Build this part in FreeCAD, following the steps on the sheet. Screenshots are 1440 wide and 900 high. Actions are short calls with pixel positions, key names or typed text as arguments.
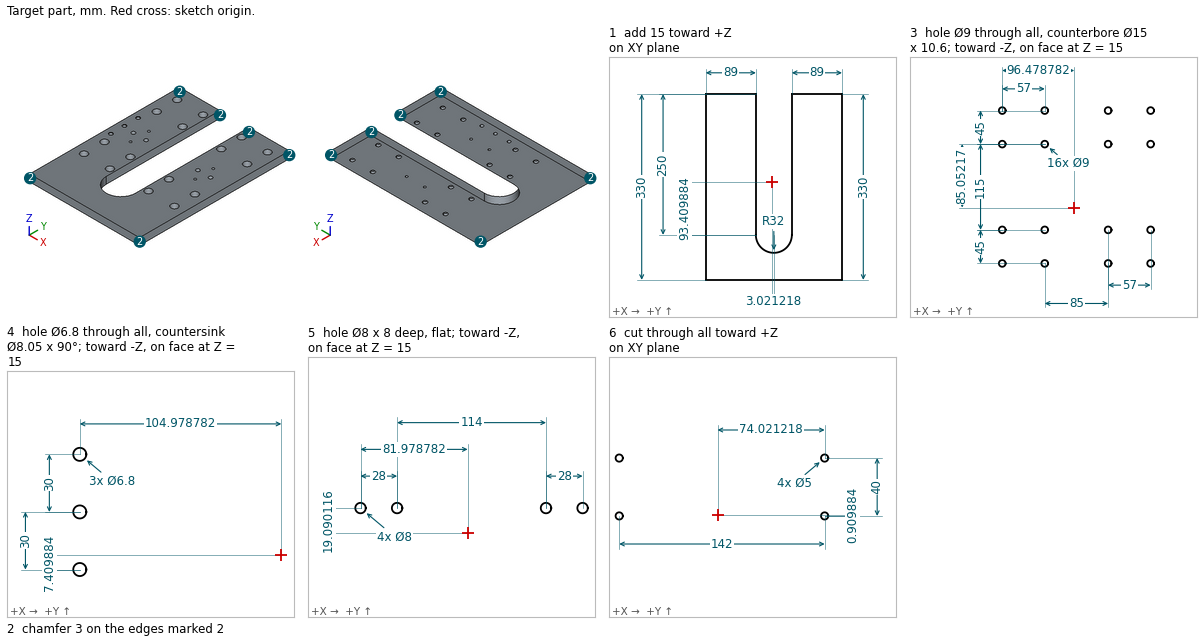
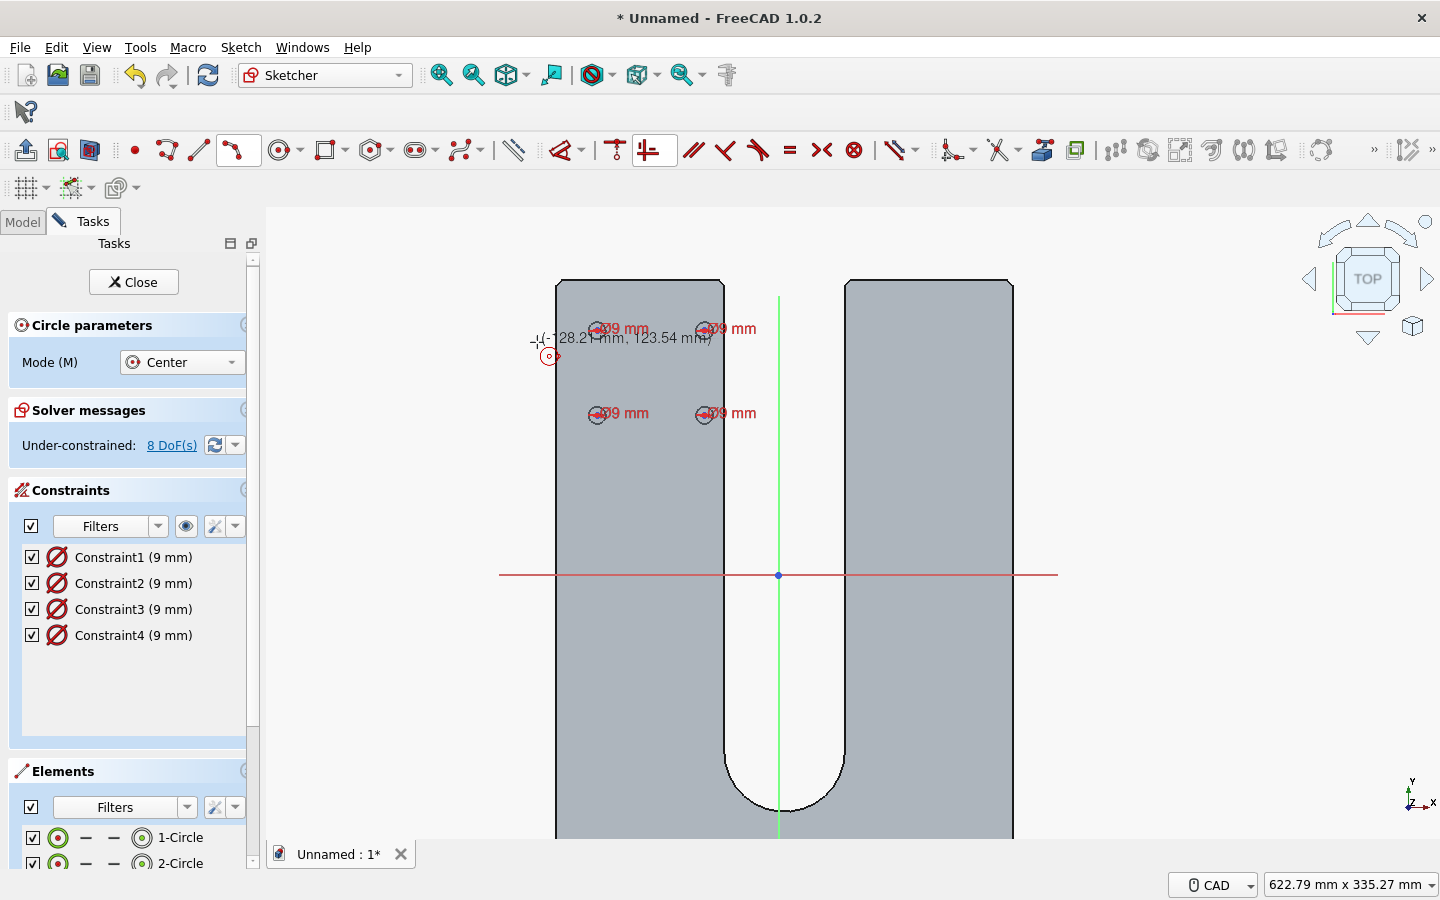
scroll(597, 632, up, 5)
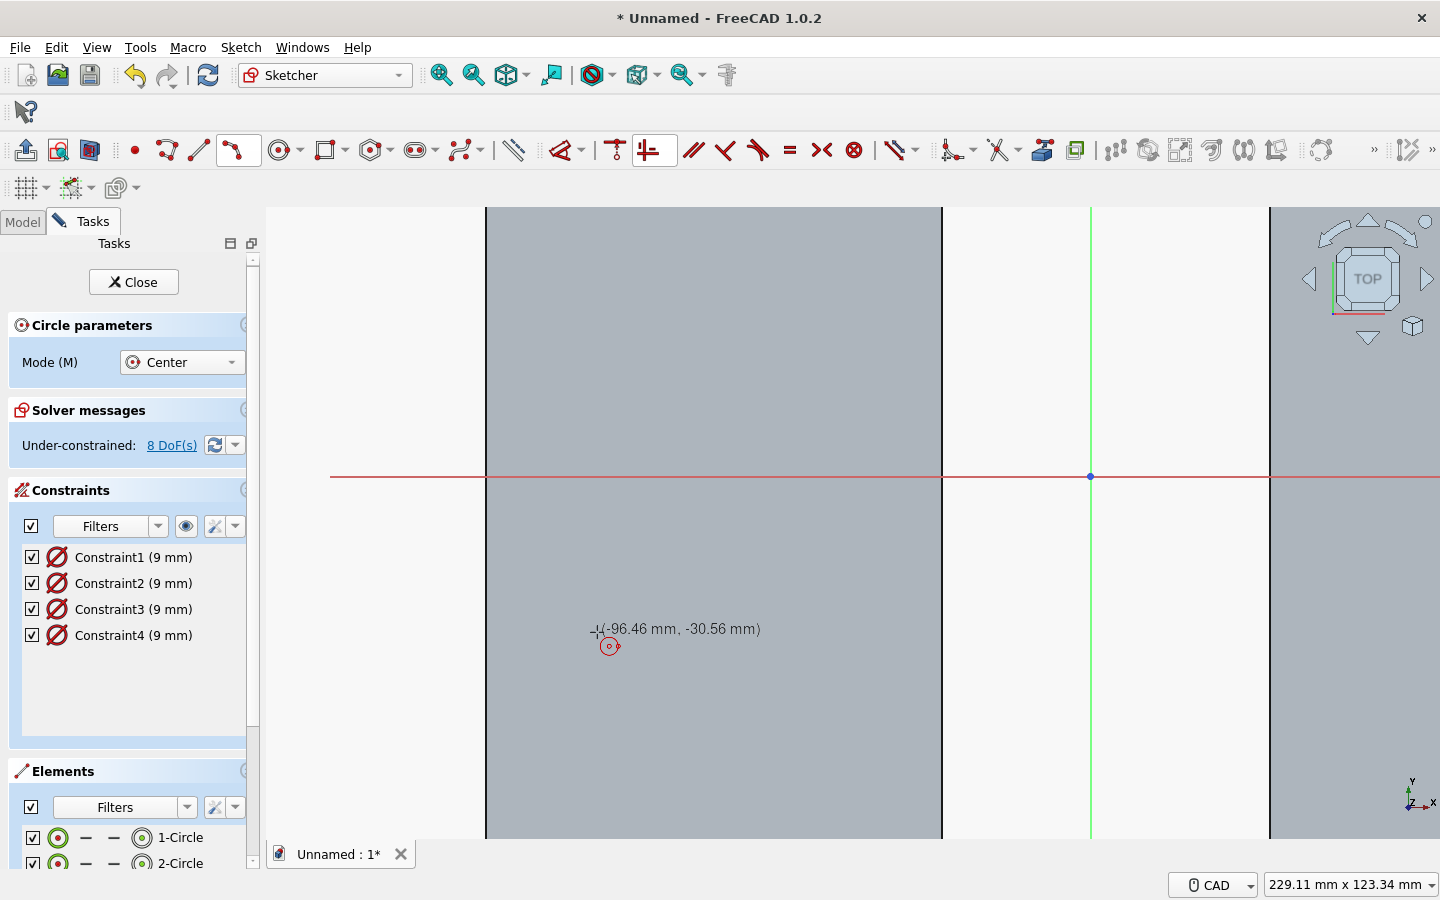
click(596, 630)
move(613, 614)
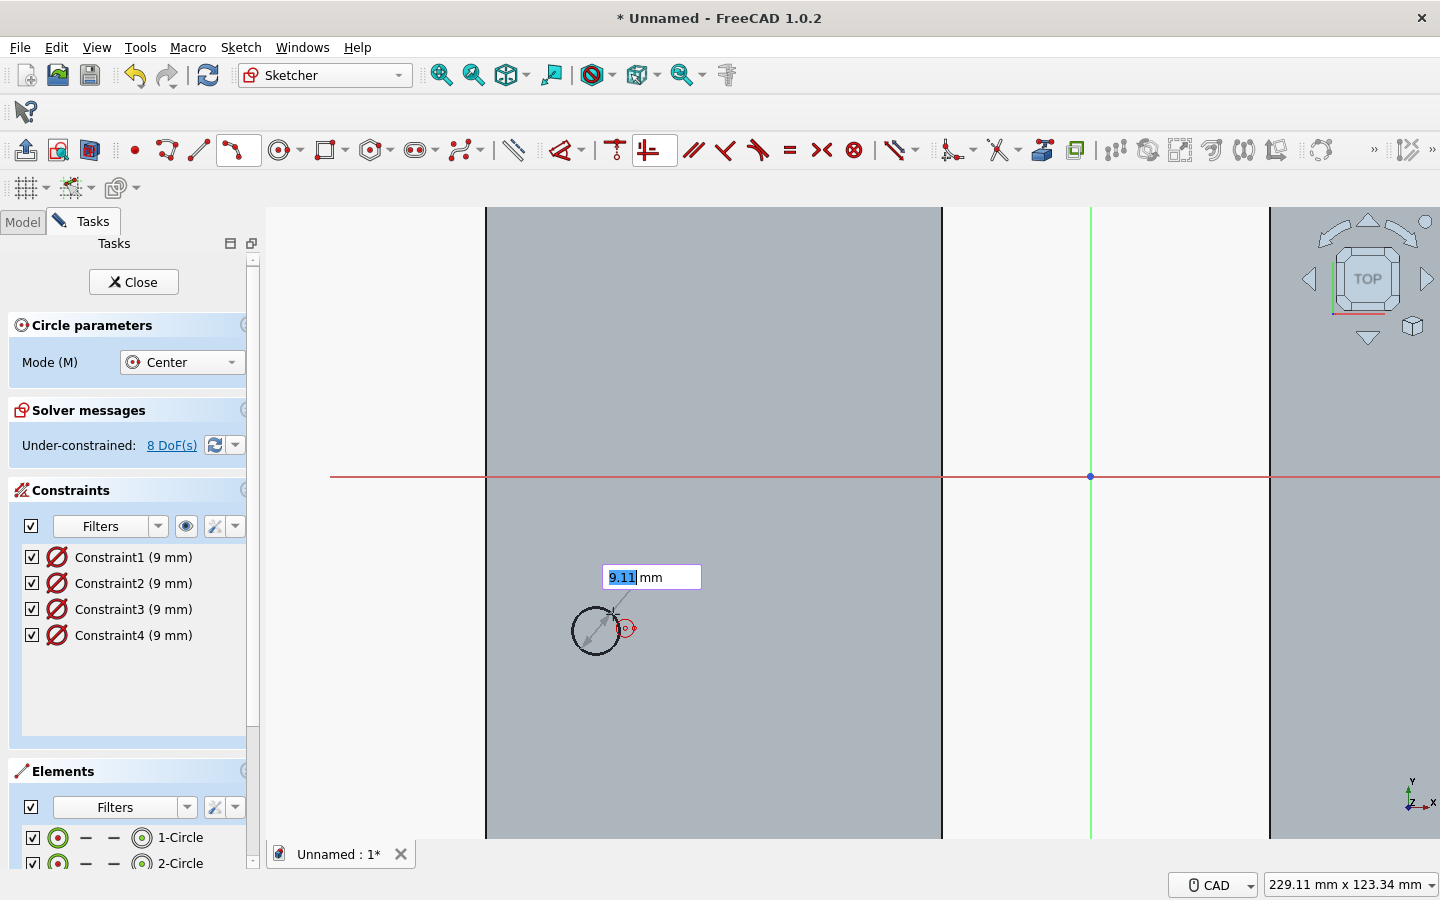
text(9)
key(Return)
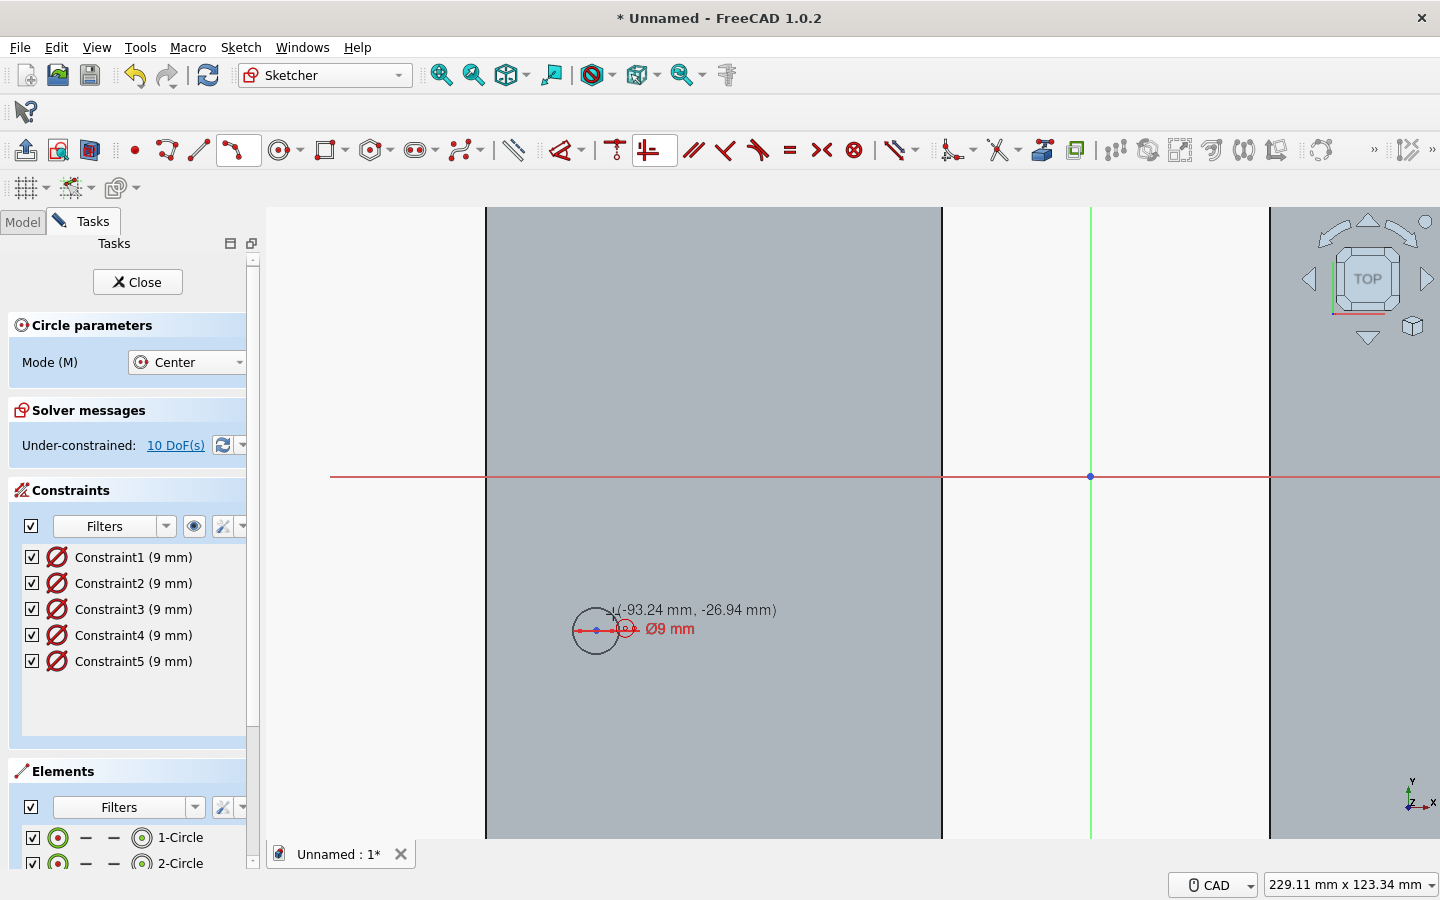
click(888, 630)
move(905, 614)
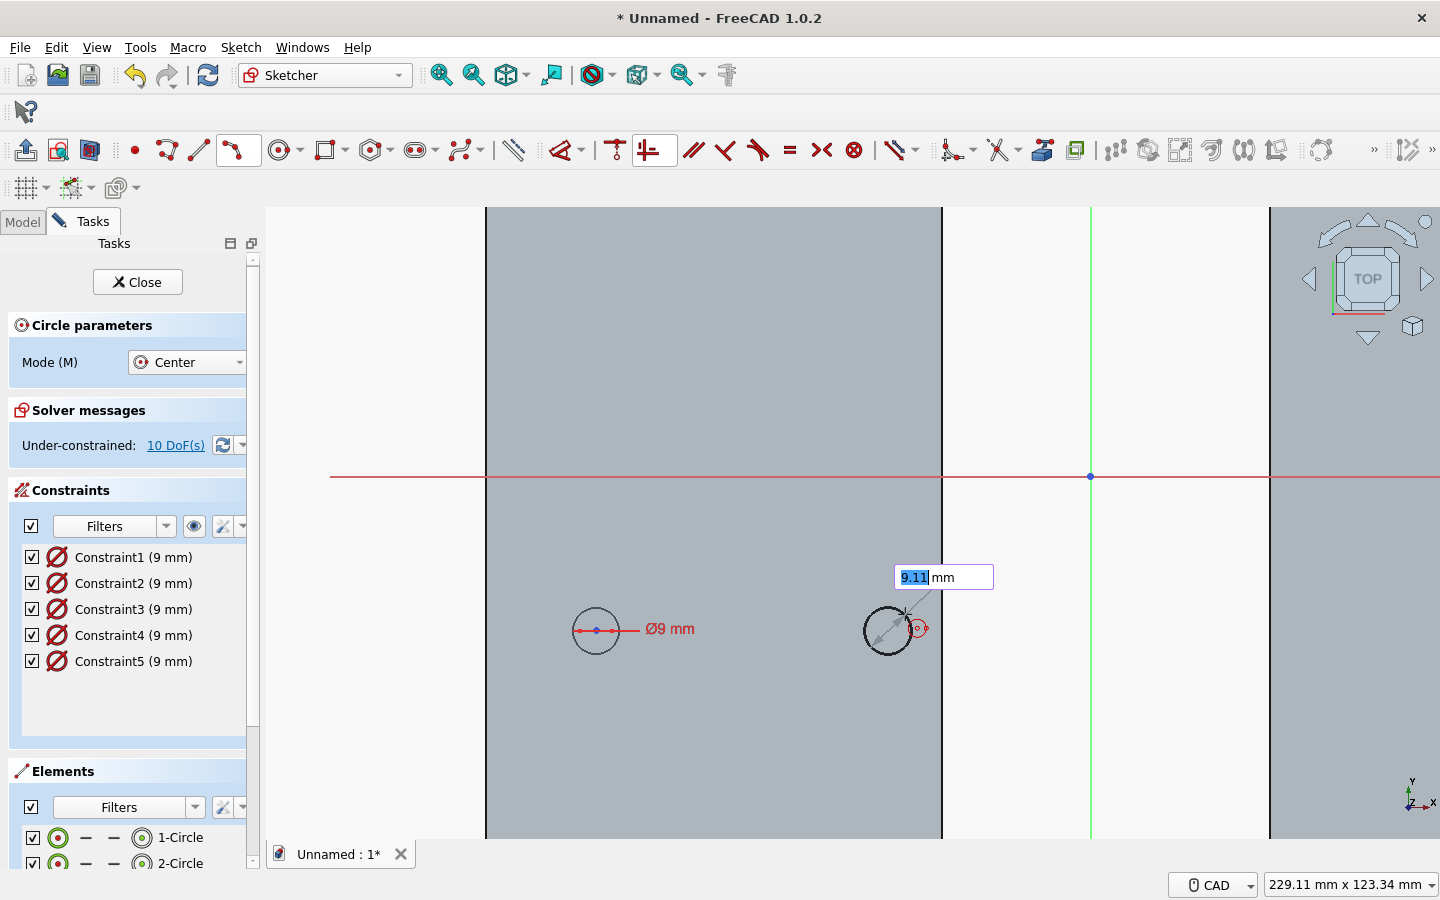
text(9)
key(Return)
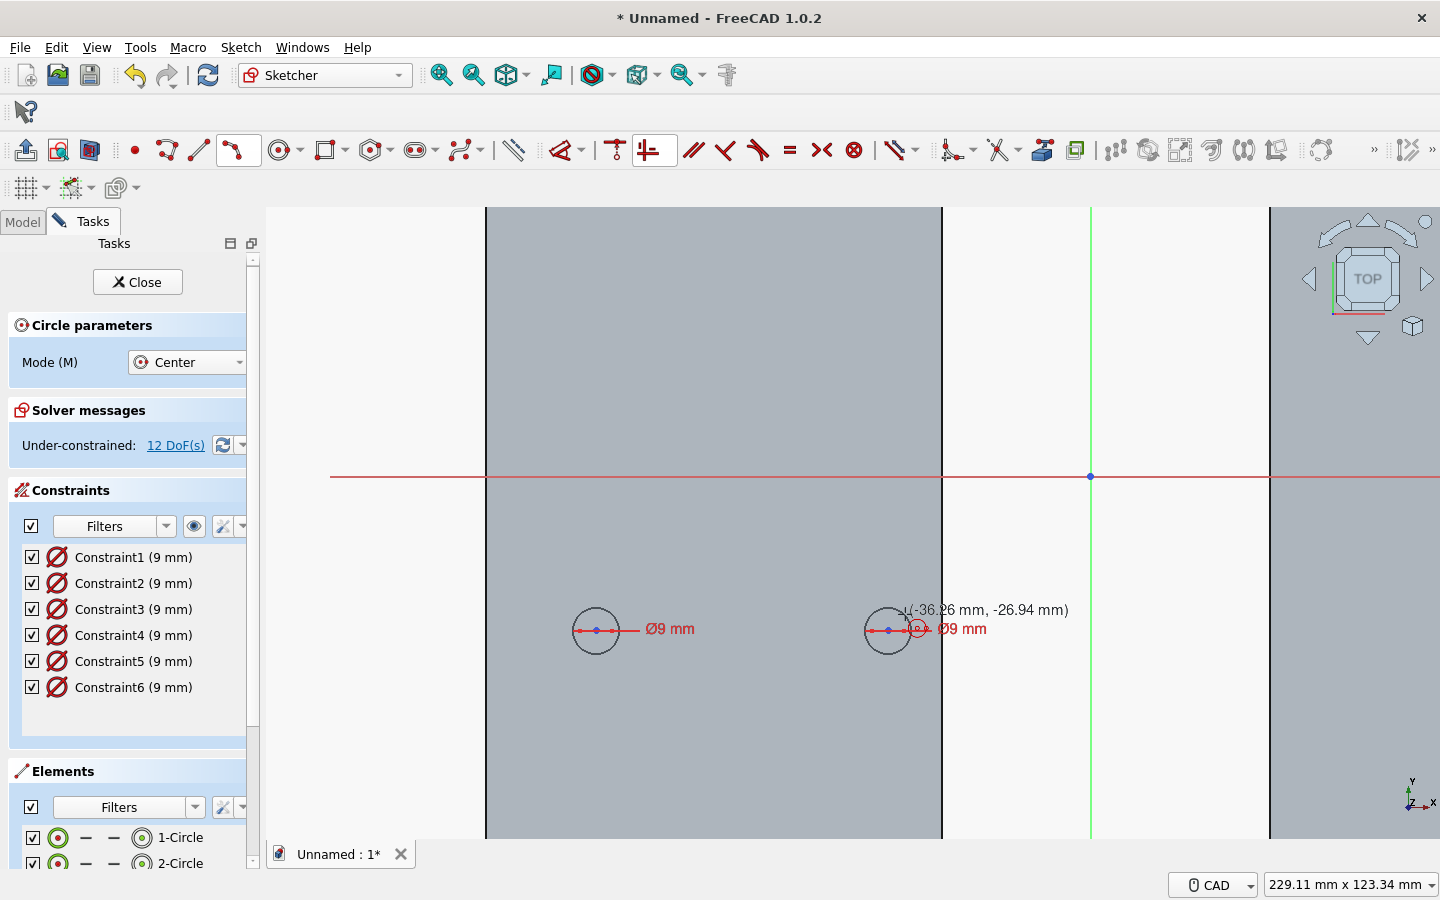
scroll(597, 632, down, 5)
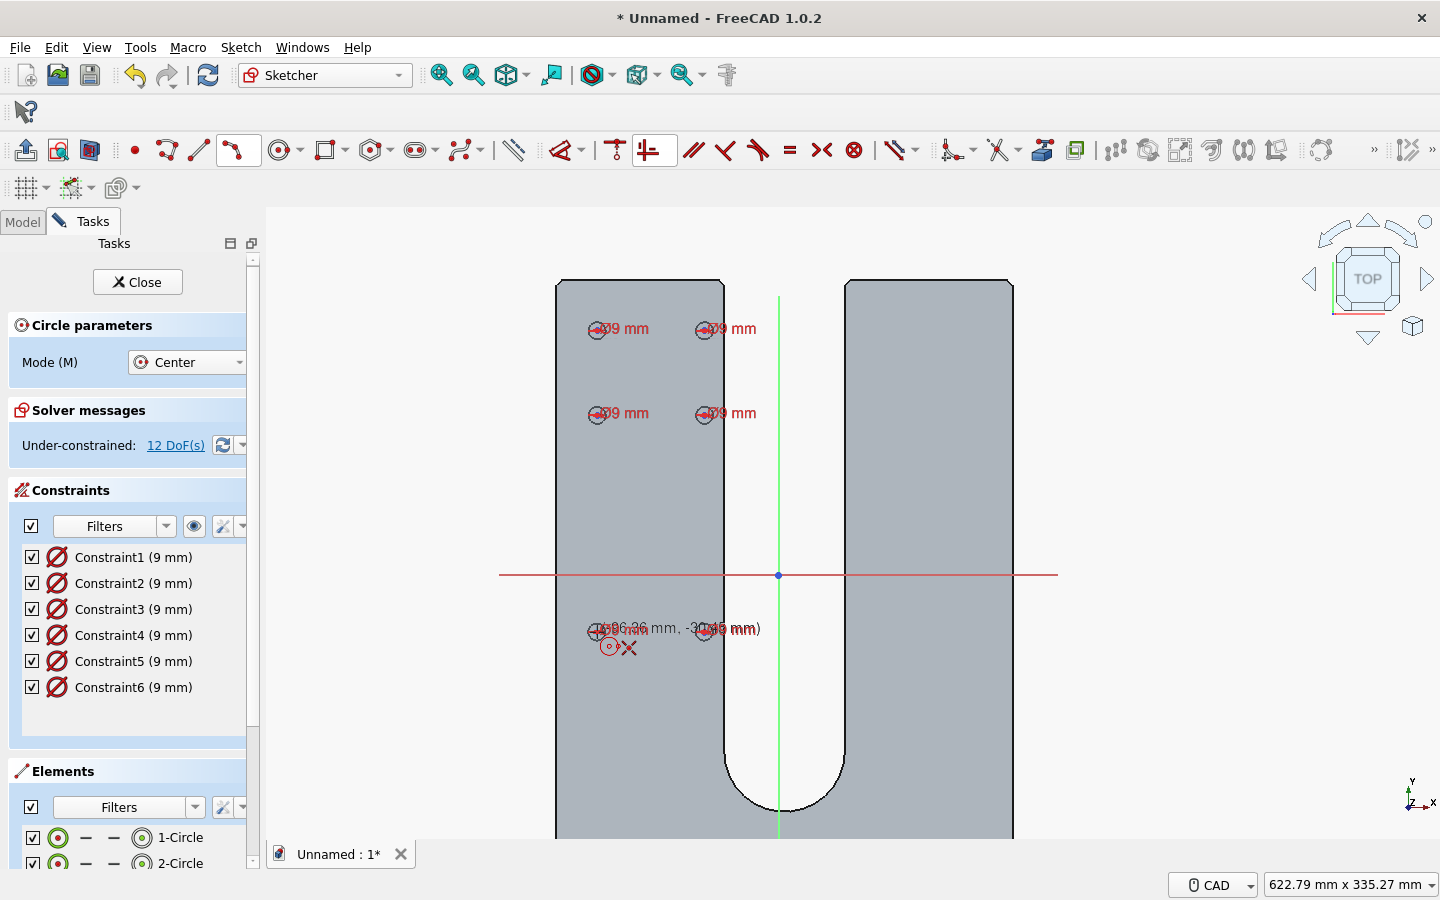
scroll(704, 717, up, 5)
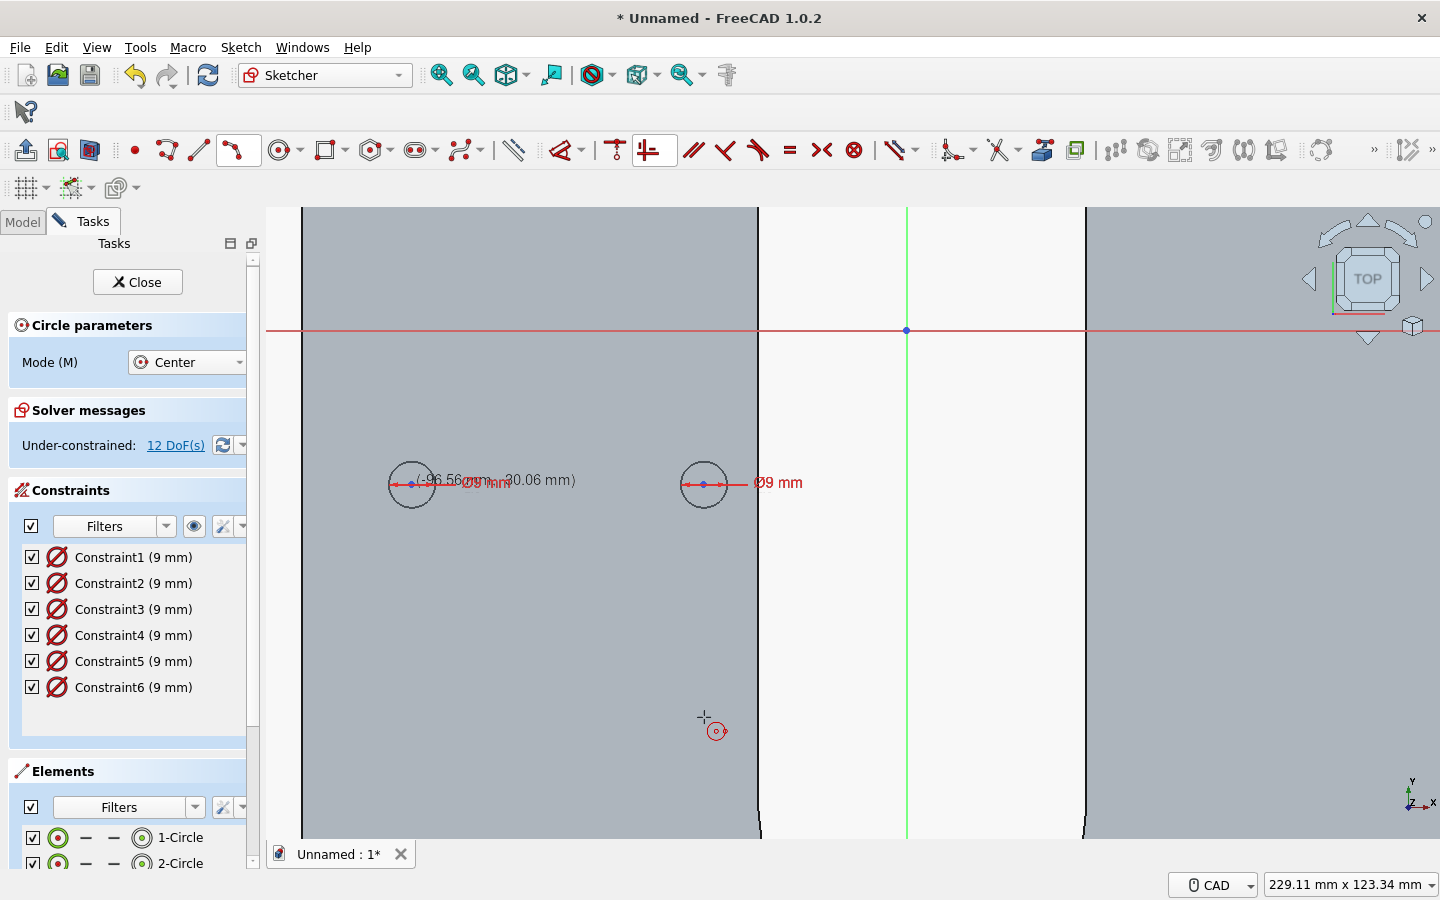
click(704, 715)
move(721, 698)